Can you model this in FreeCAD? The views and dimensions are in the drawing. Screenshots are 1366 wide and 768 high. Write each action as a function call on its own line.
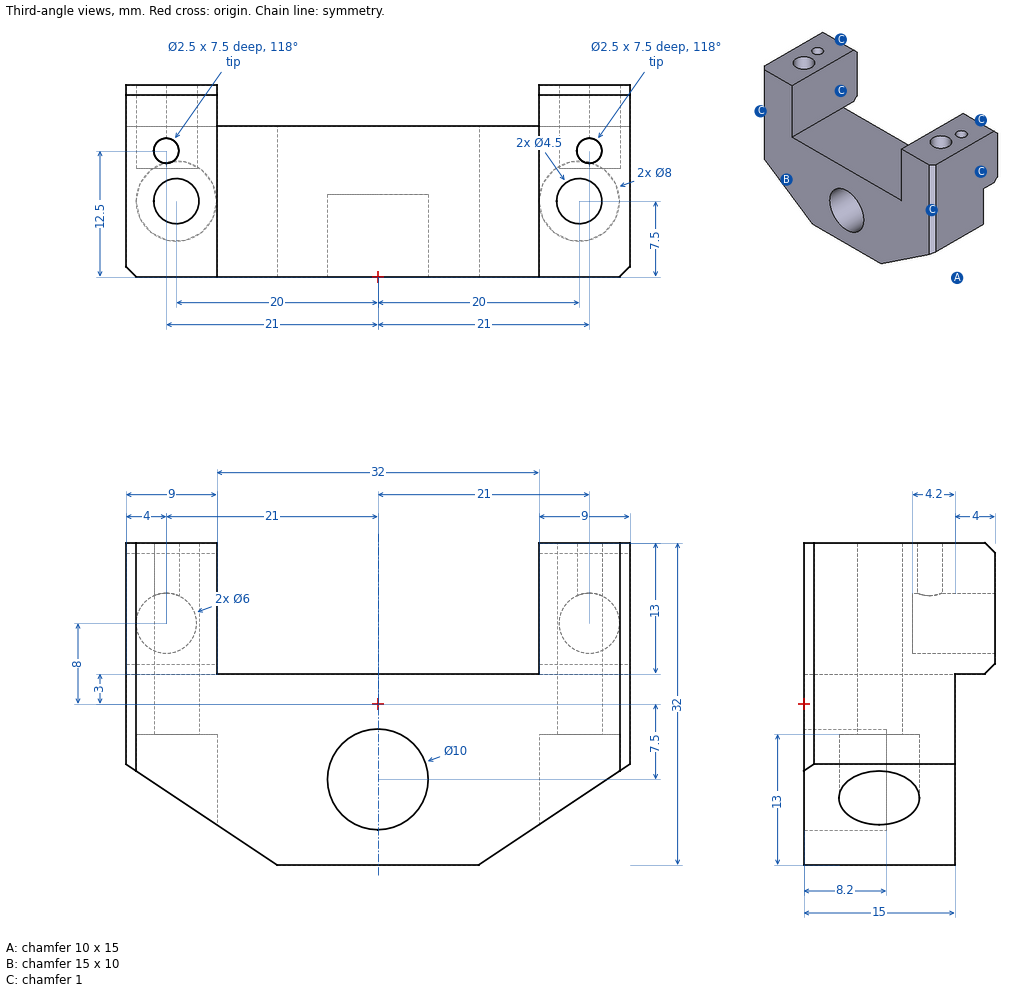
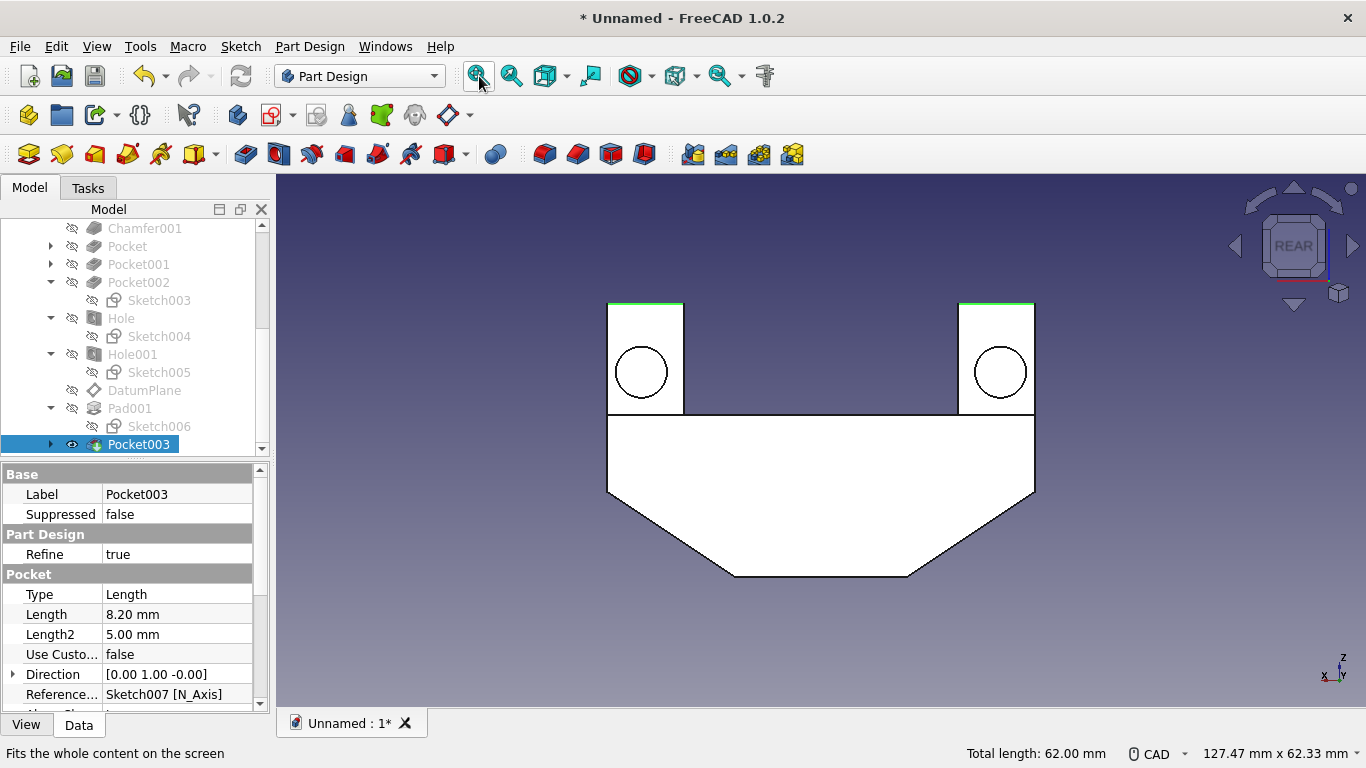
click(996, 414, ctrl)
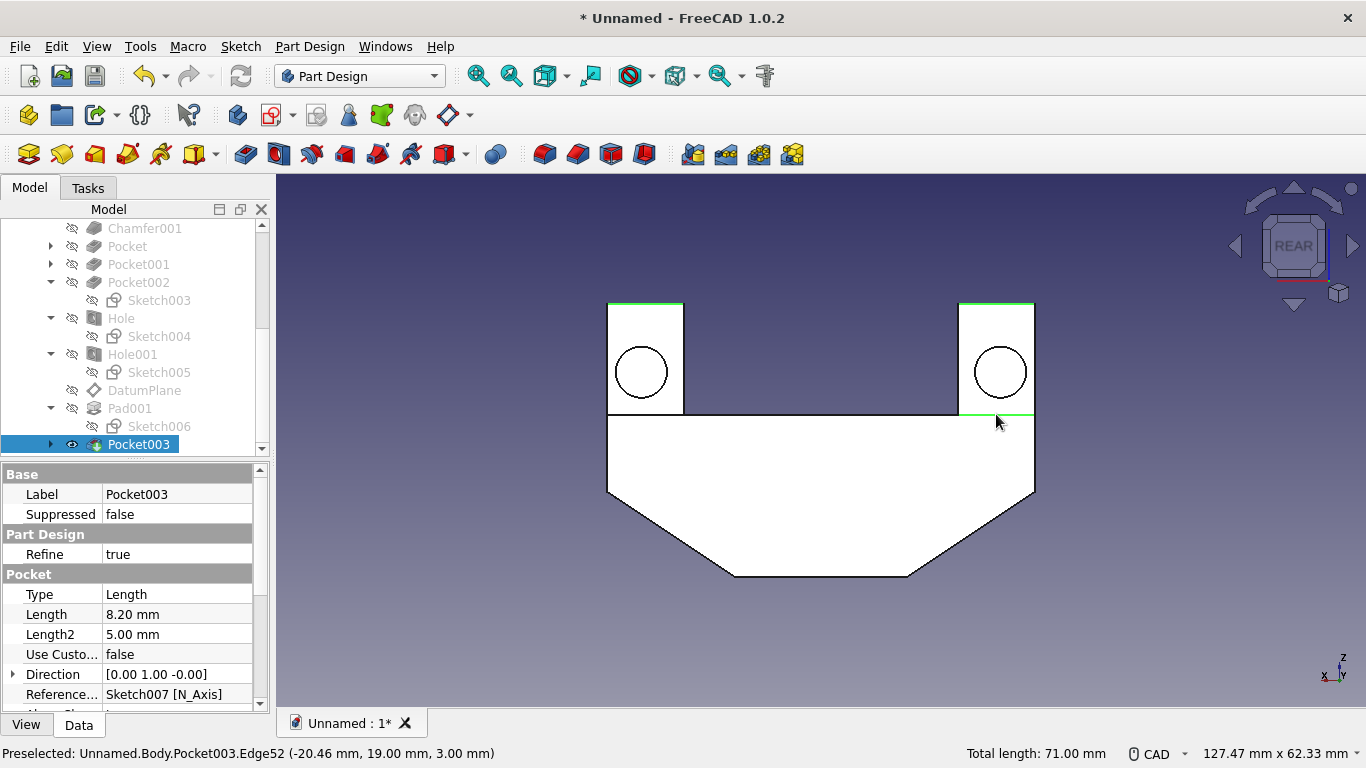
click(646, 414, ctrl)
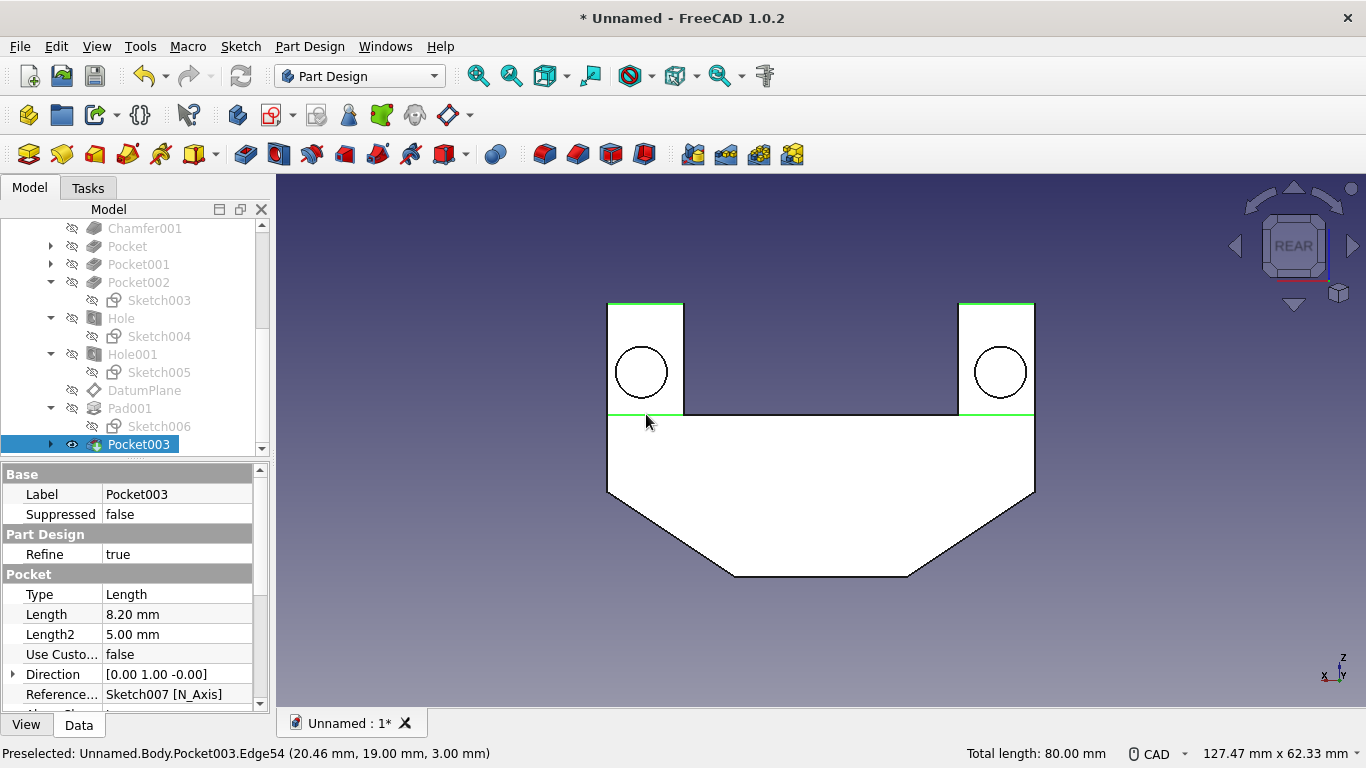
click(578, 154)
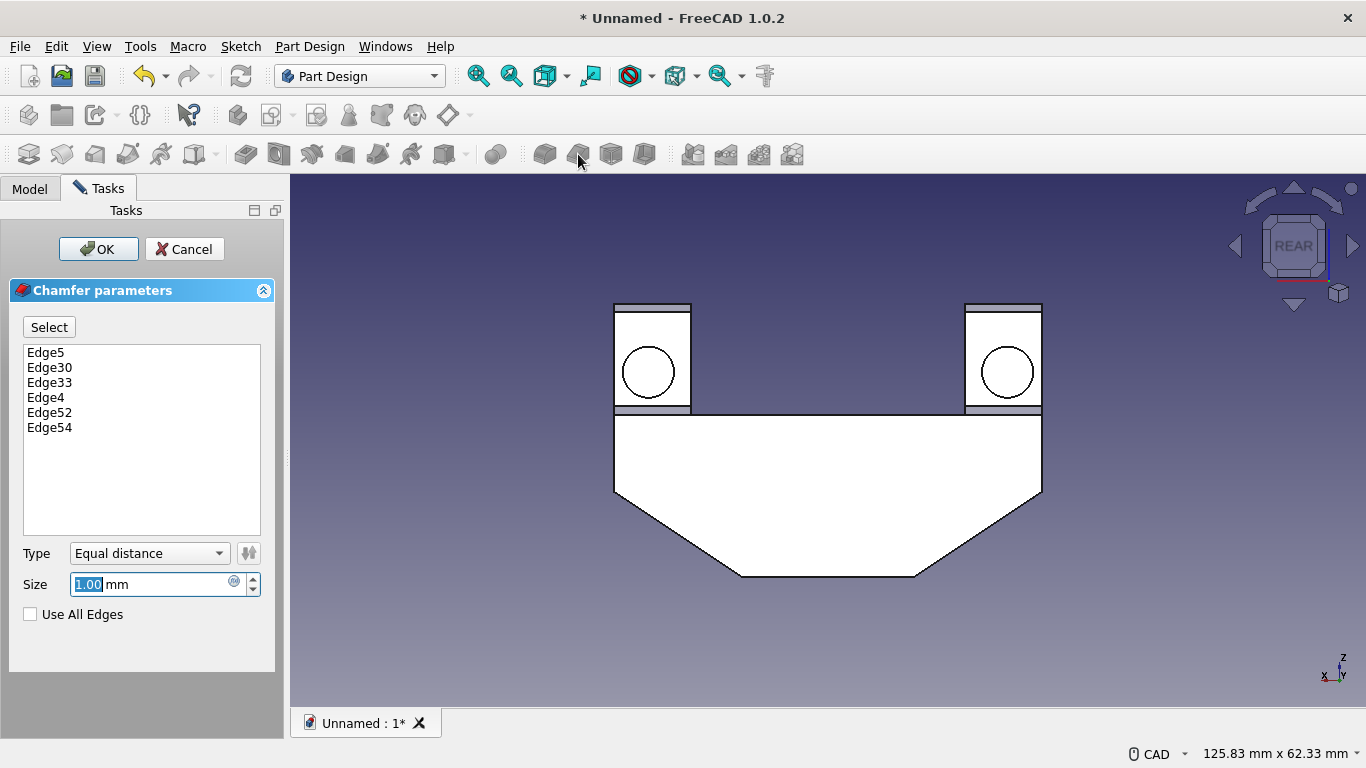
text(1)
key(Tab)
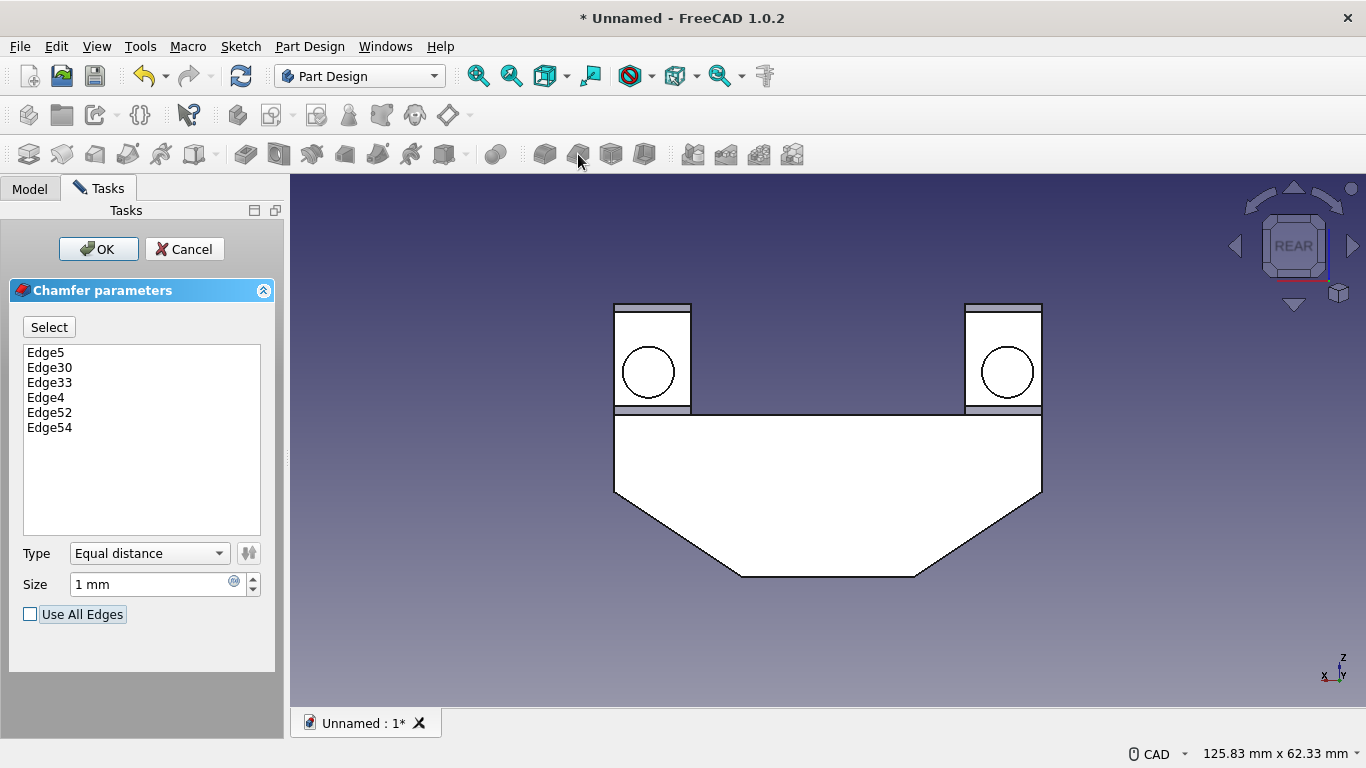
click(99, 249)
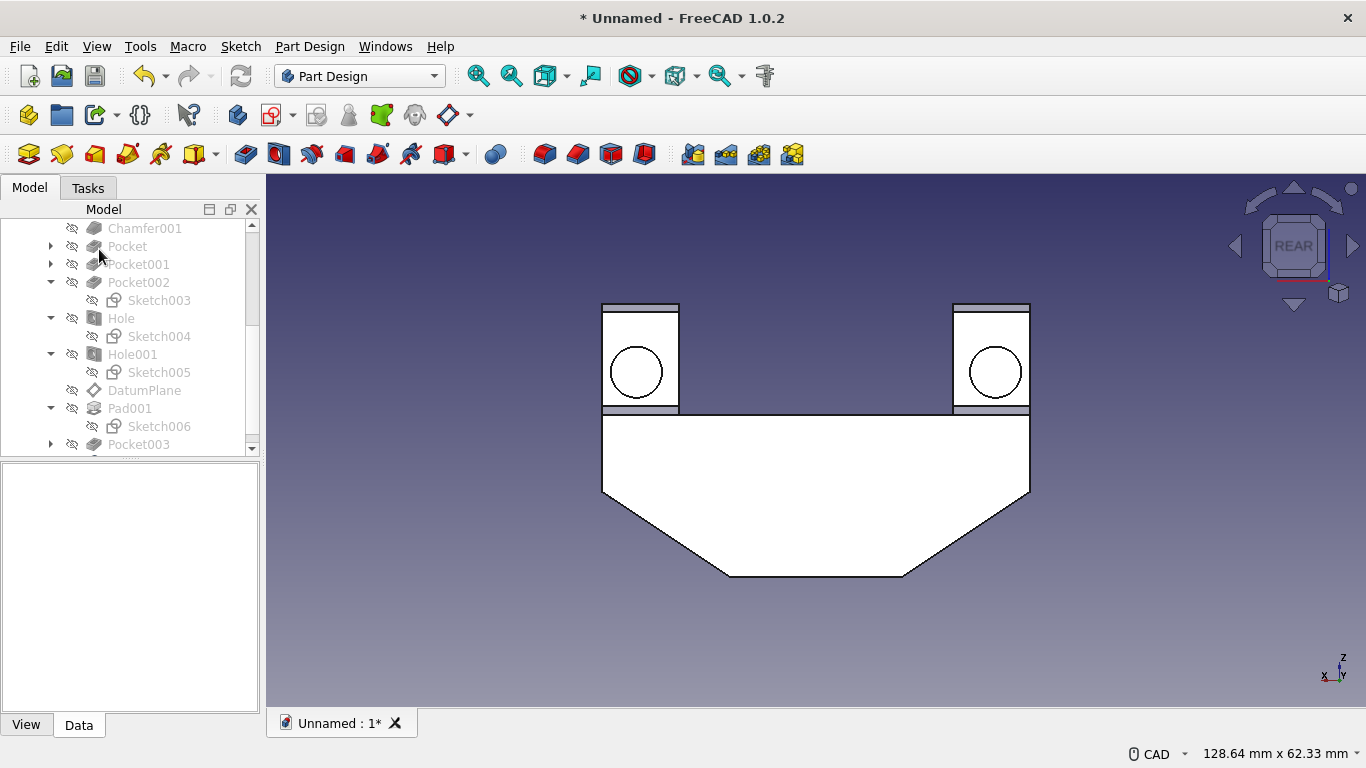
key(0)